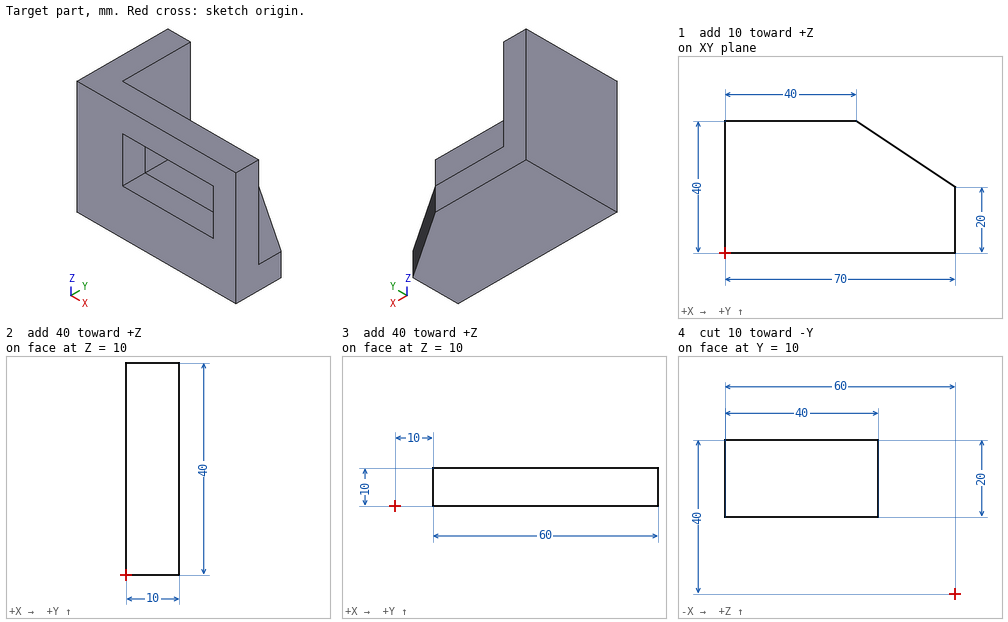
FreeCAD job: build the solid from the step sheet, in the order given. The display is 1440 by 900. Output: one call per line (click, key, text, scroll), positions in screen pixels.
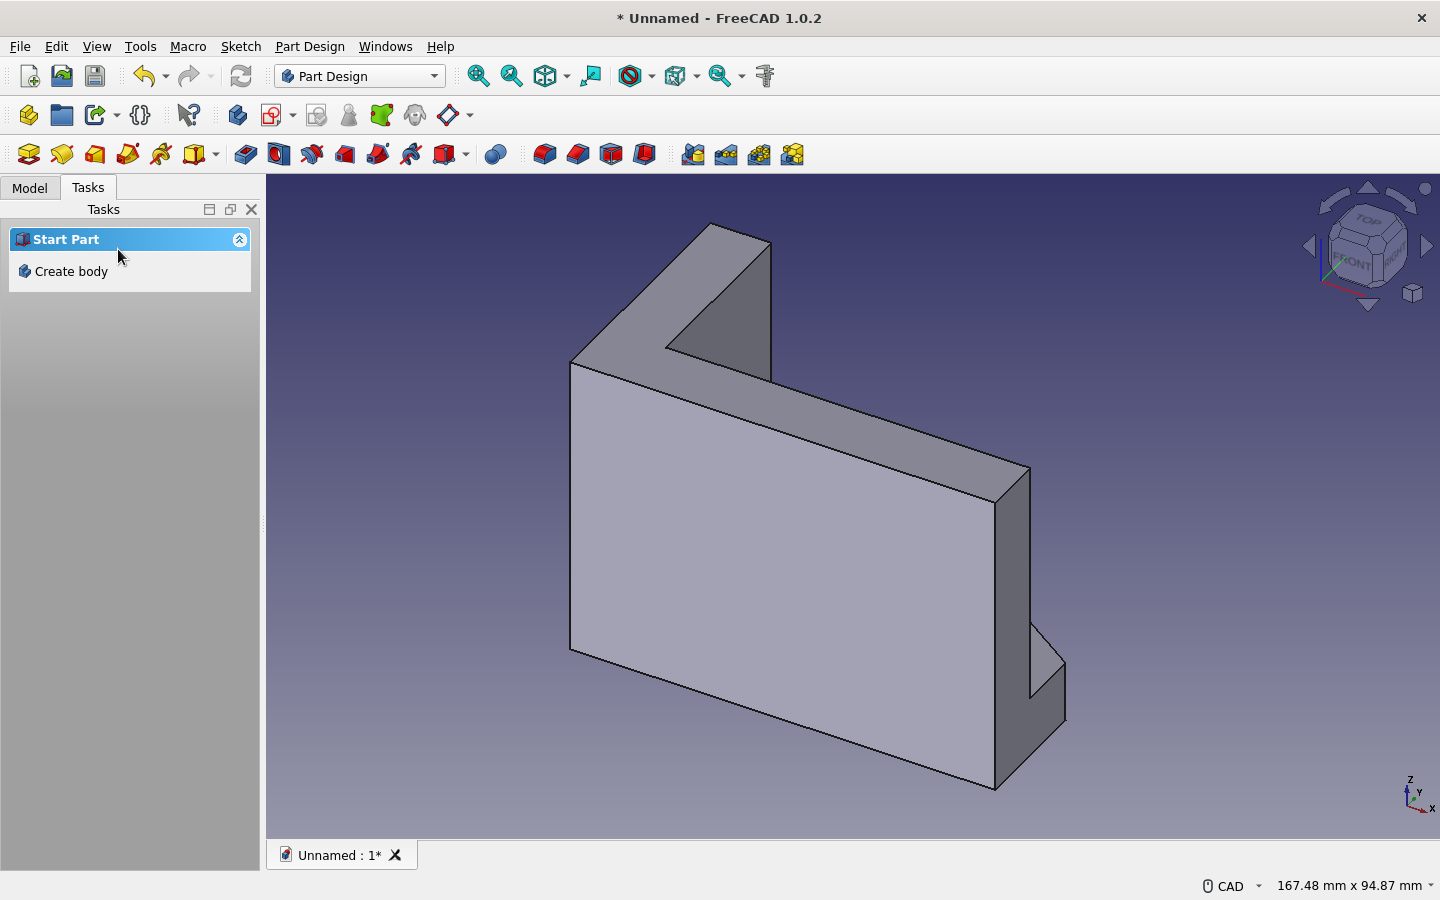
key(4)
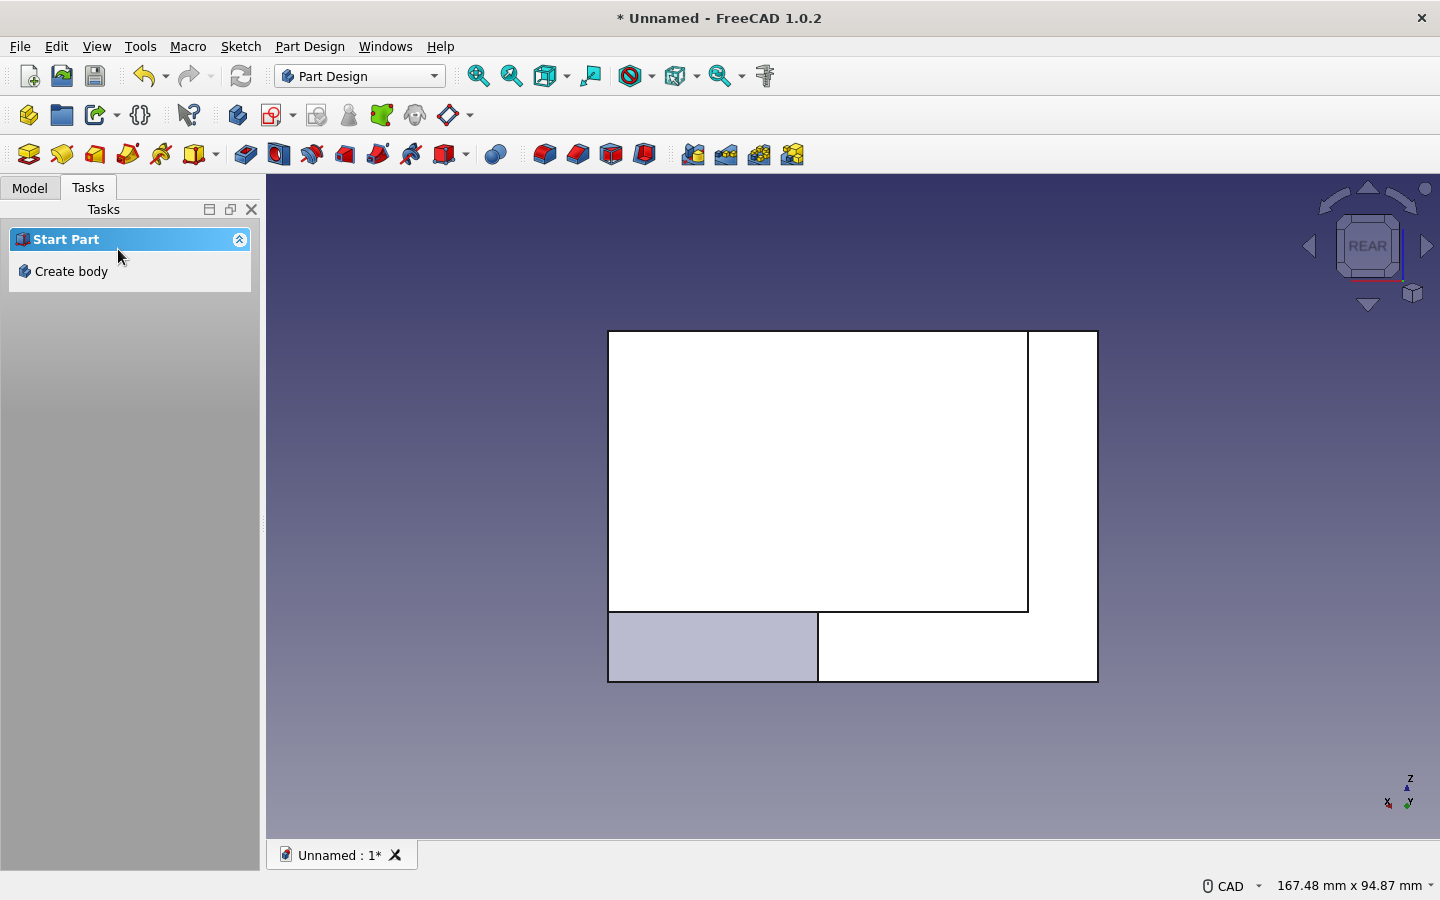
click(758, 470)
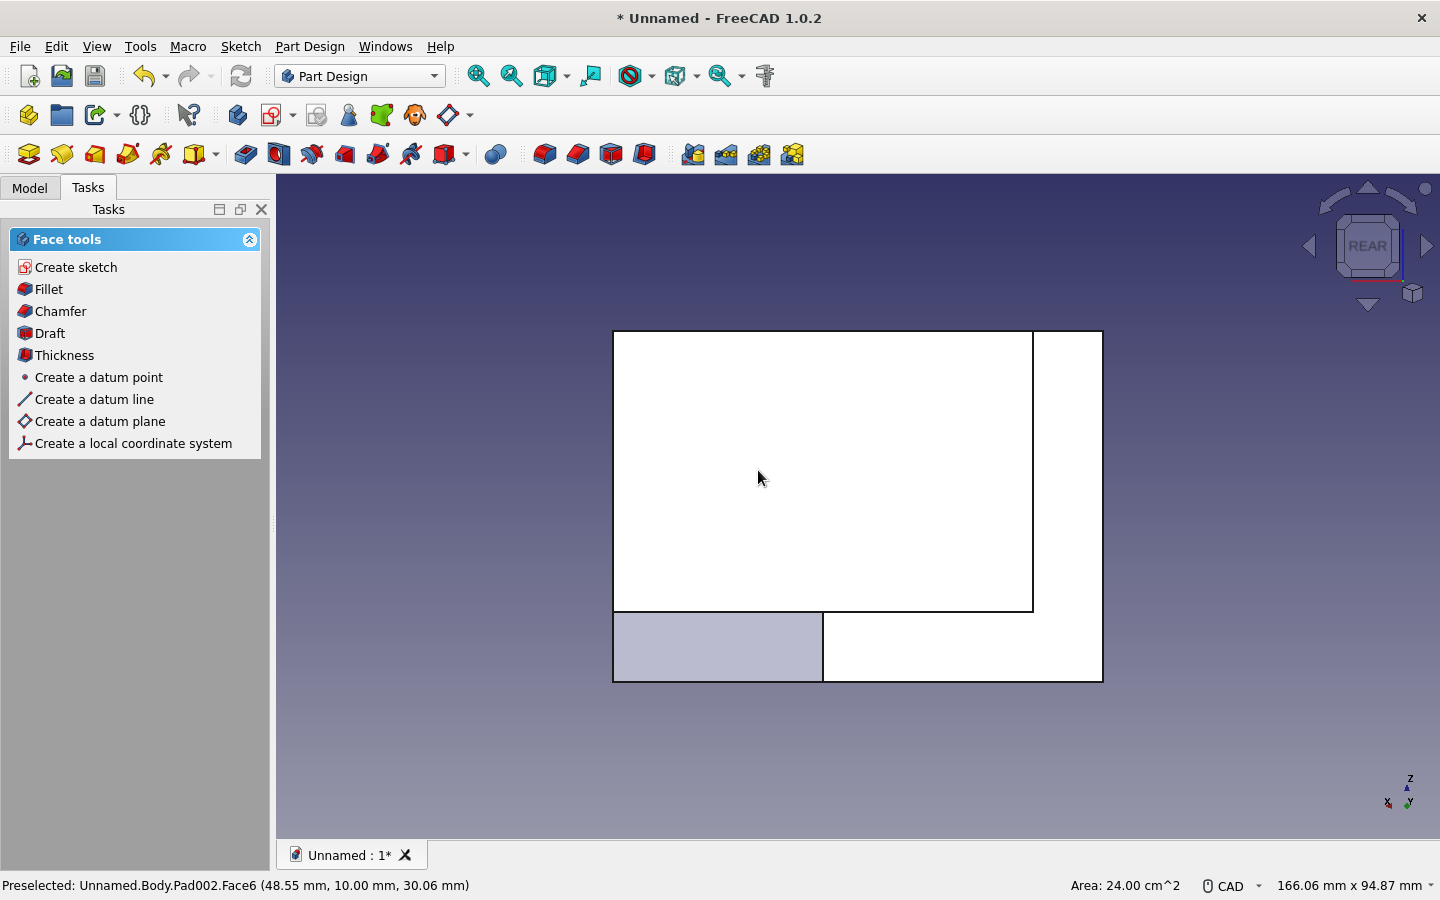
click(270, 116)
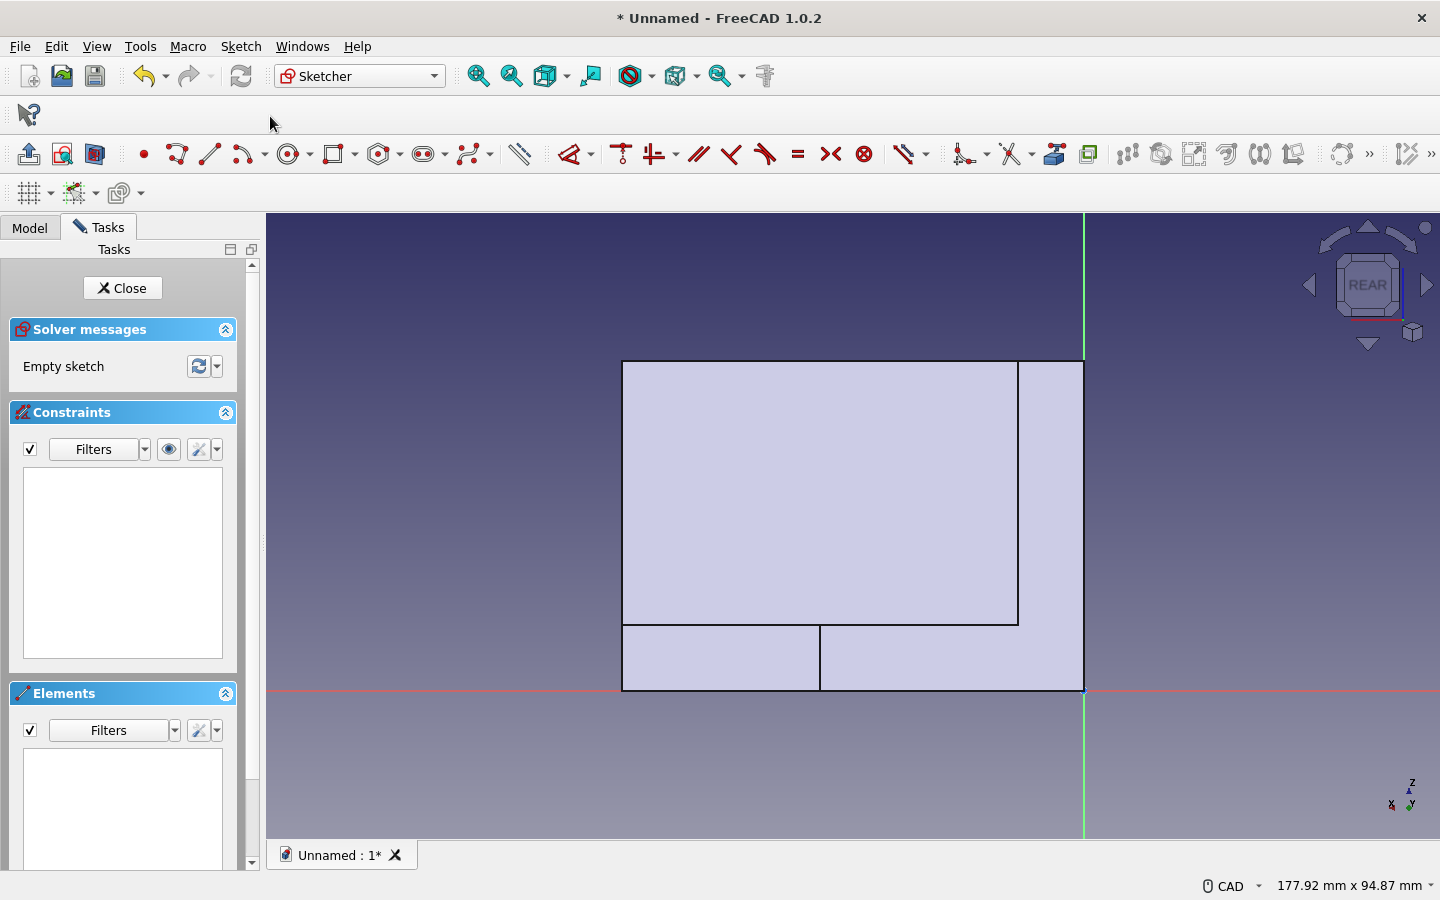
key(q)
key(s)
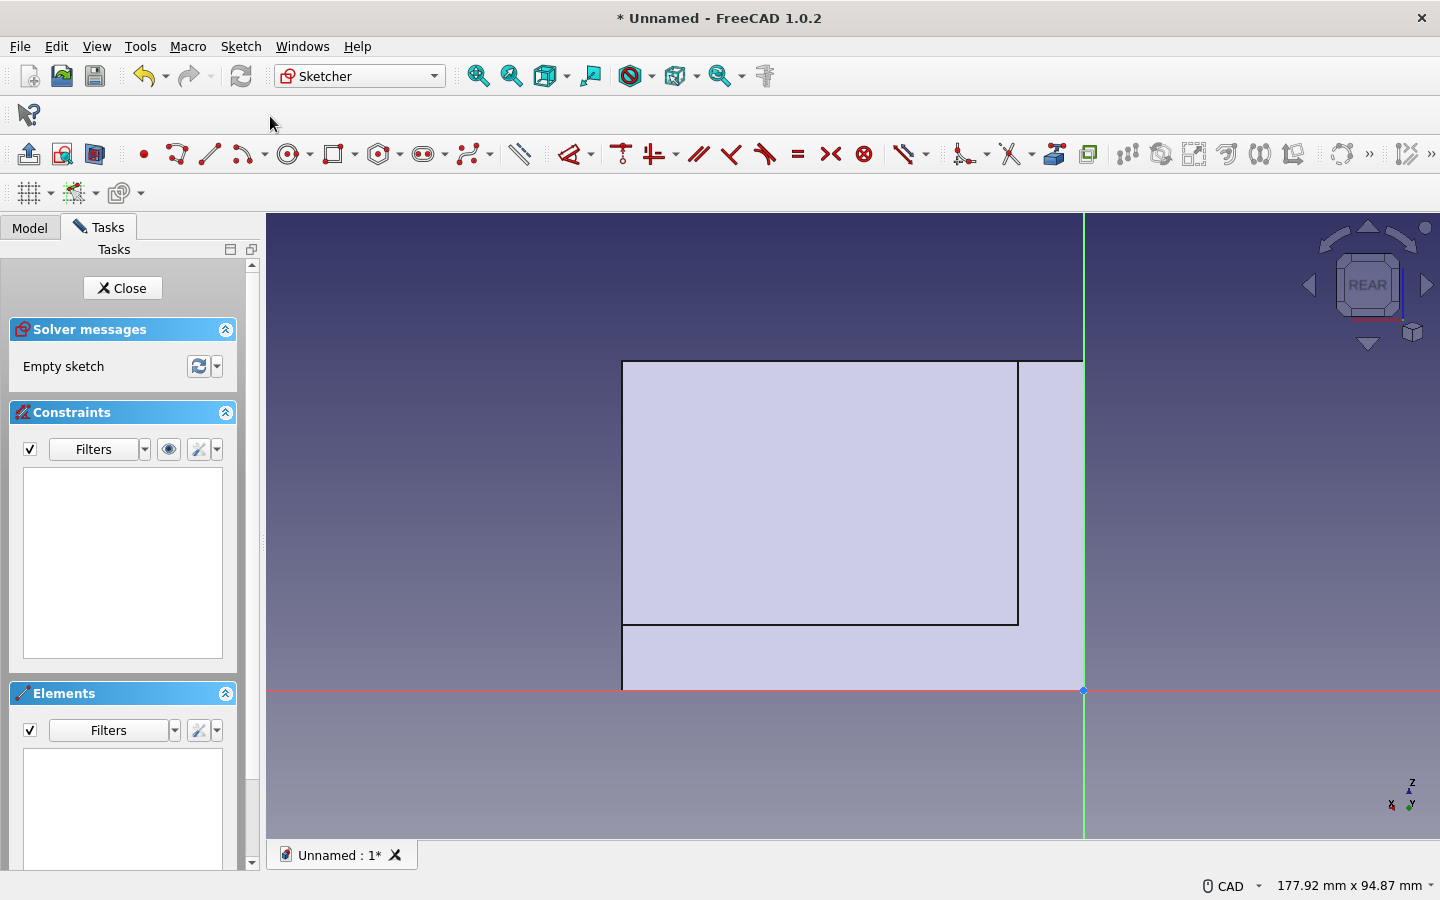
scroll(1092, 626, up, 2)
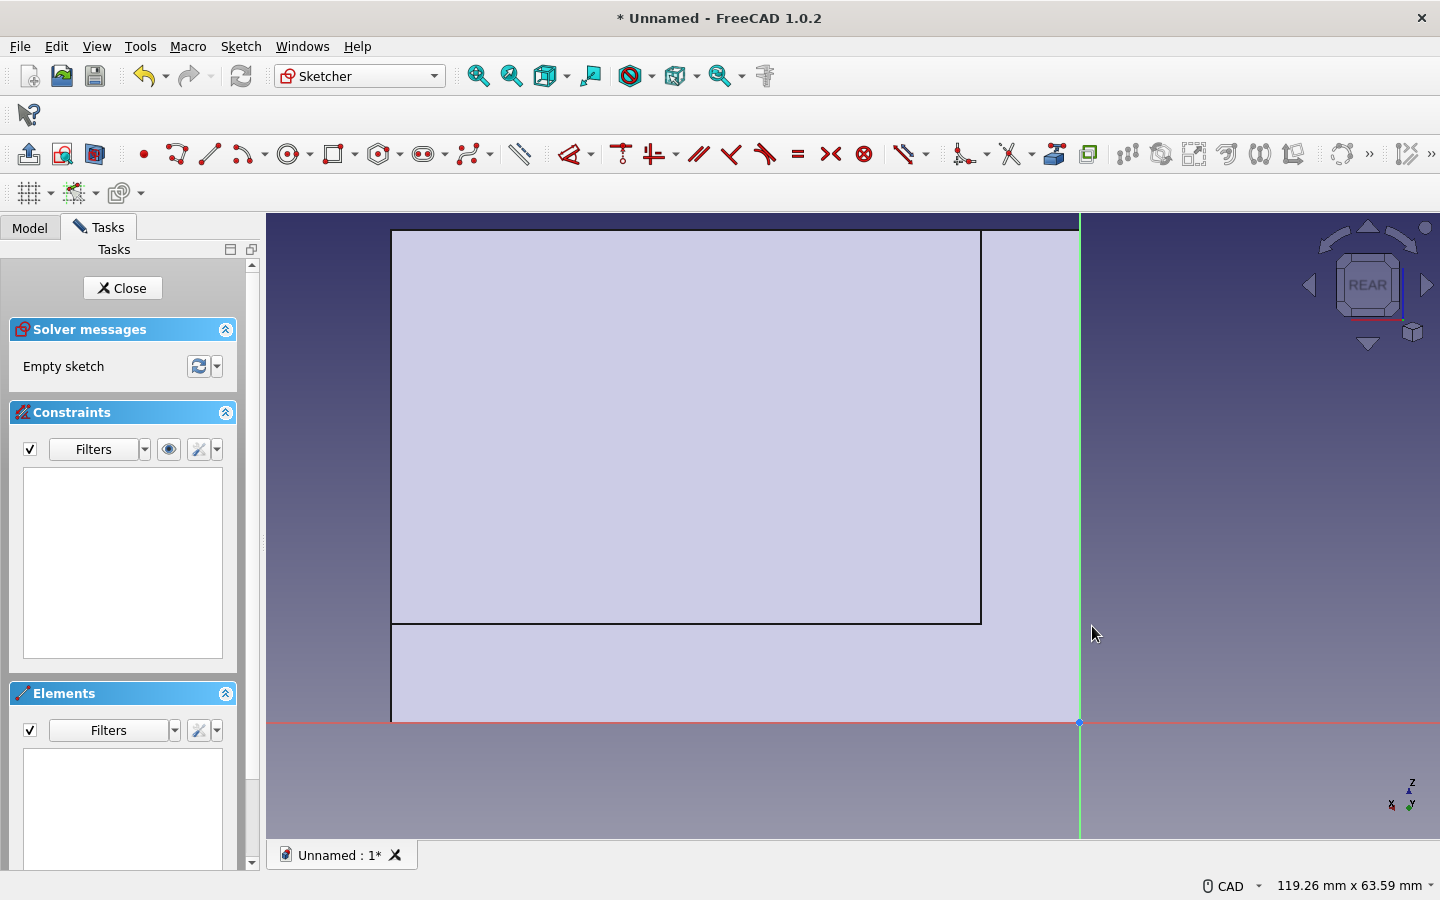
click(332, 154)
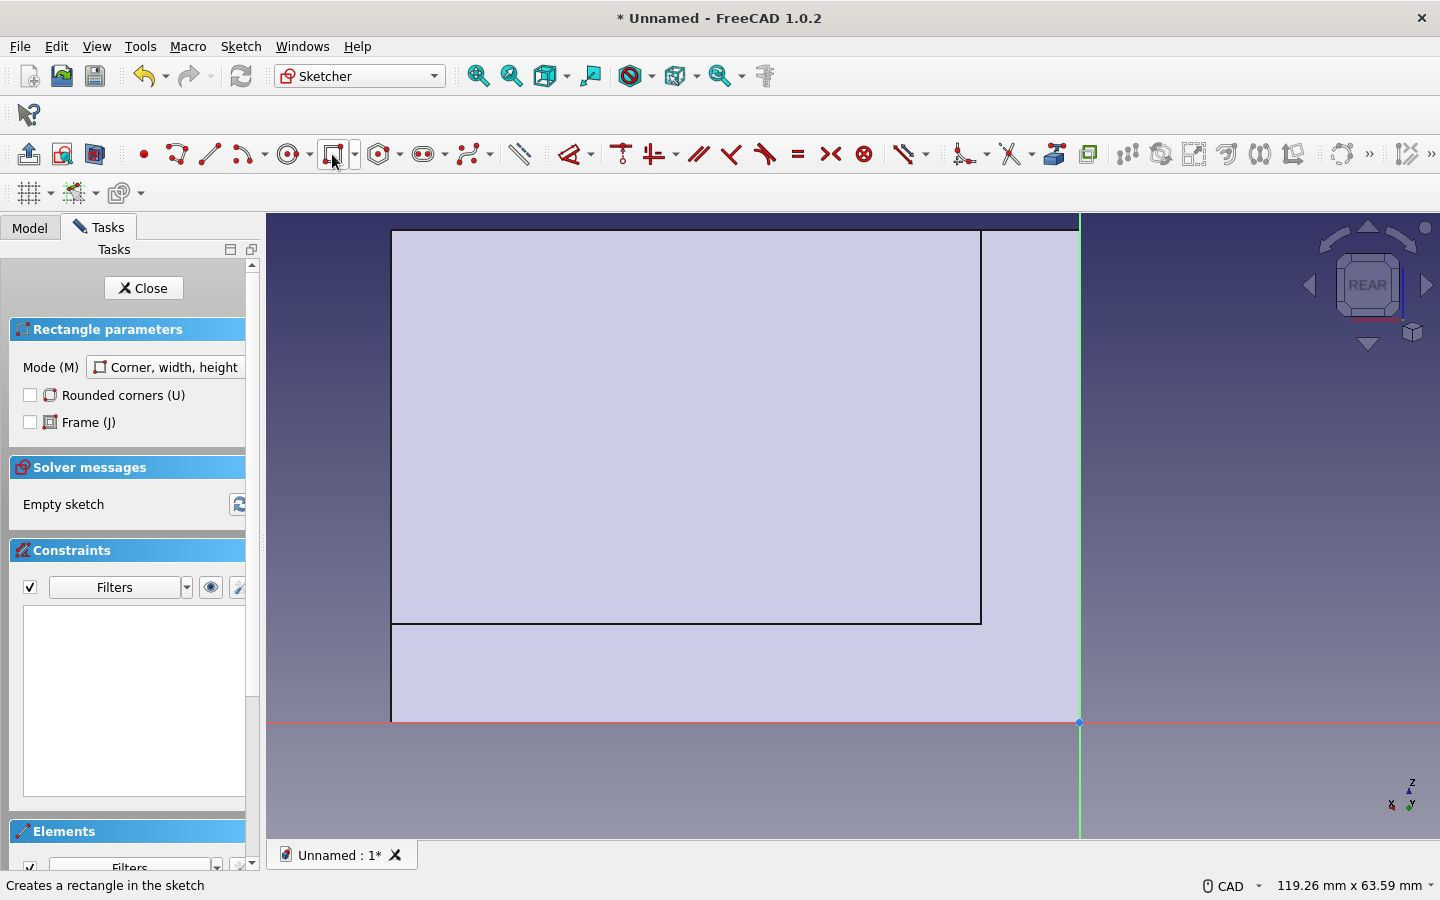
click(489, 329)
move(883, 526)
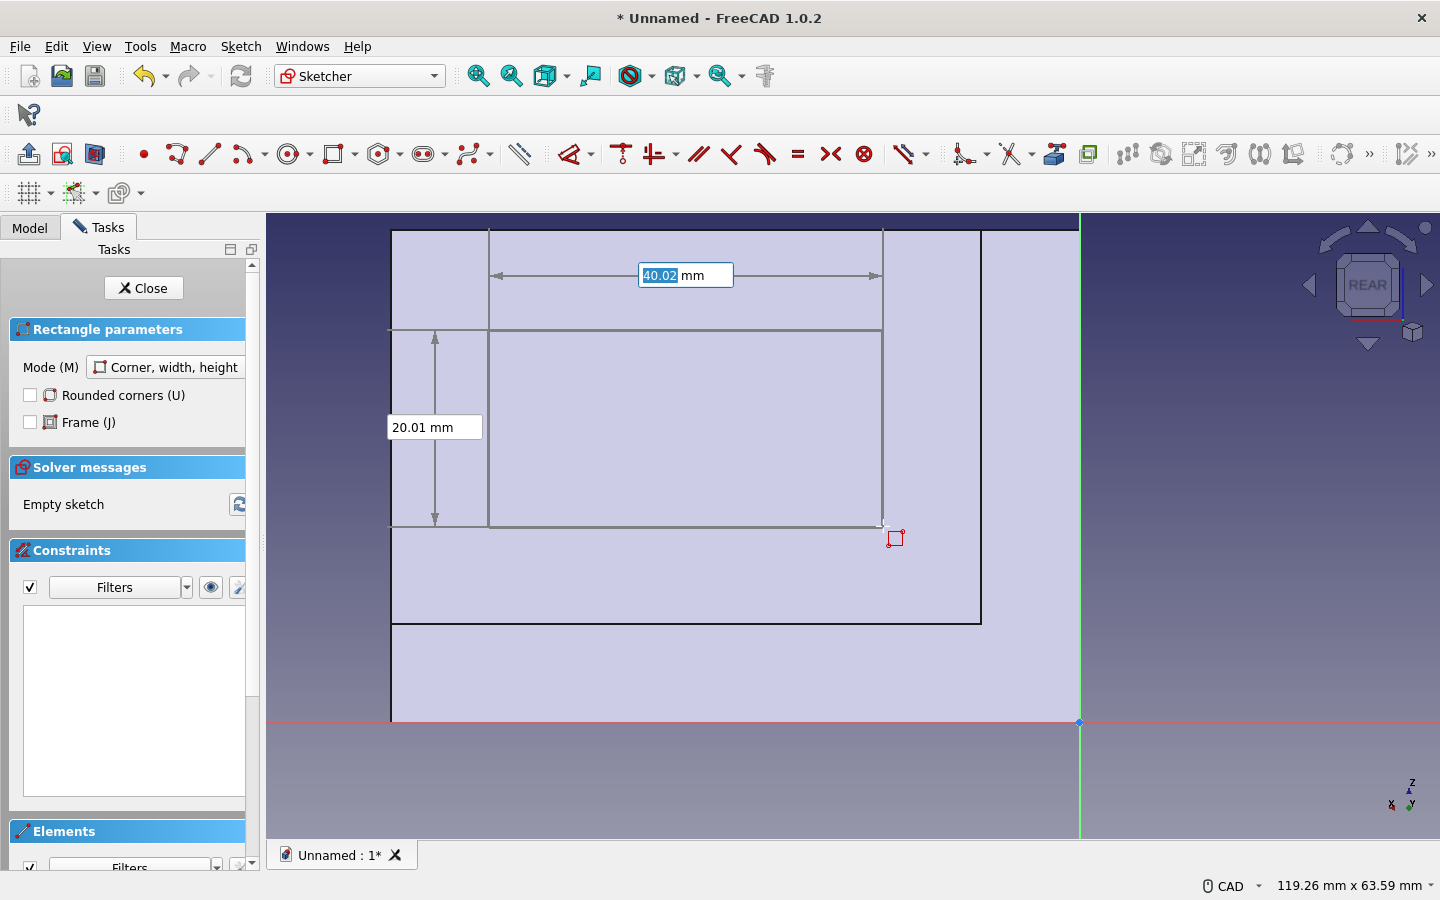
text(40)
key(Tab)
text(20)
key(Return)
key(Escape)